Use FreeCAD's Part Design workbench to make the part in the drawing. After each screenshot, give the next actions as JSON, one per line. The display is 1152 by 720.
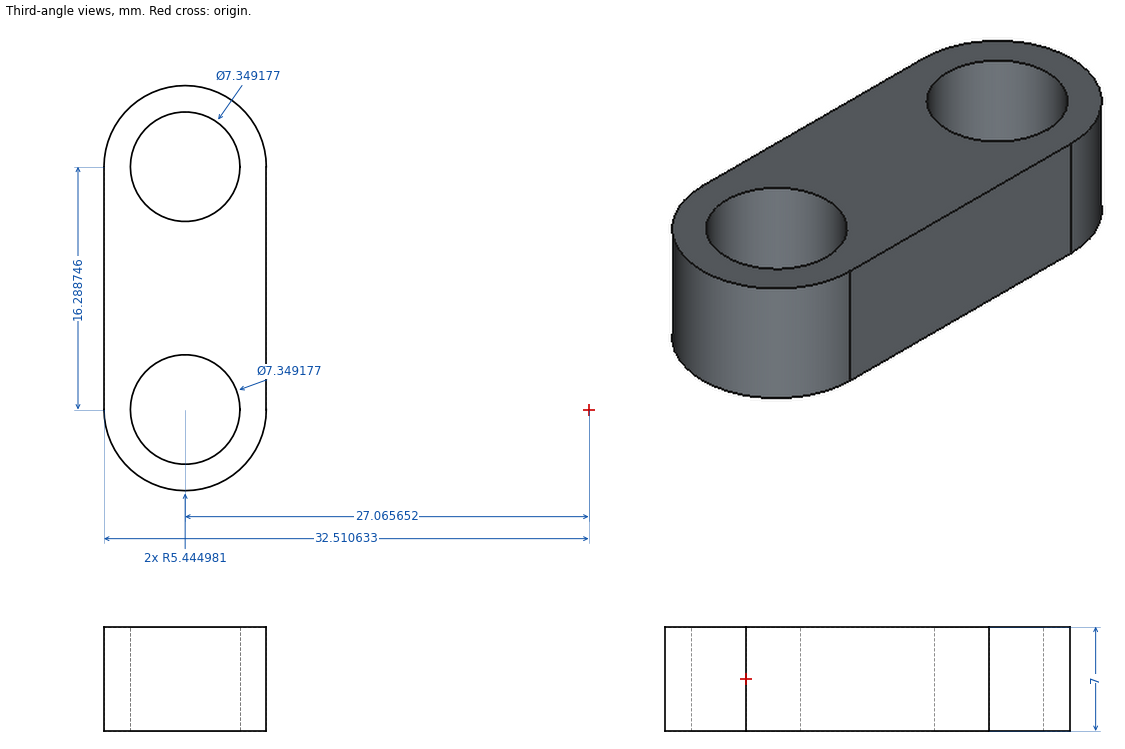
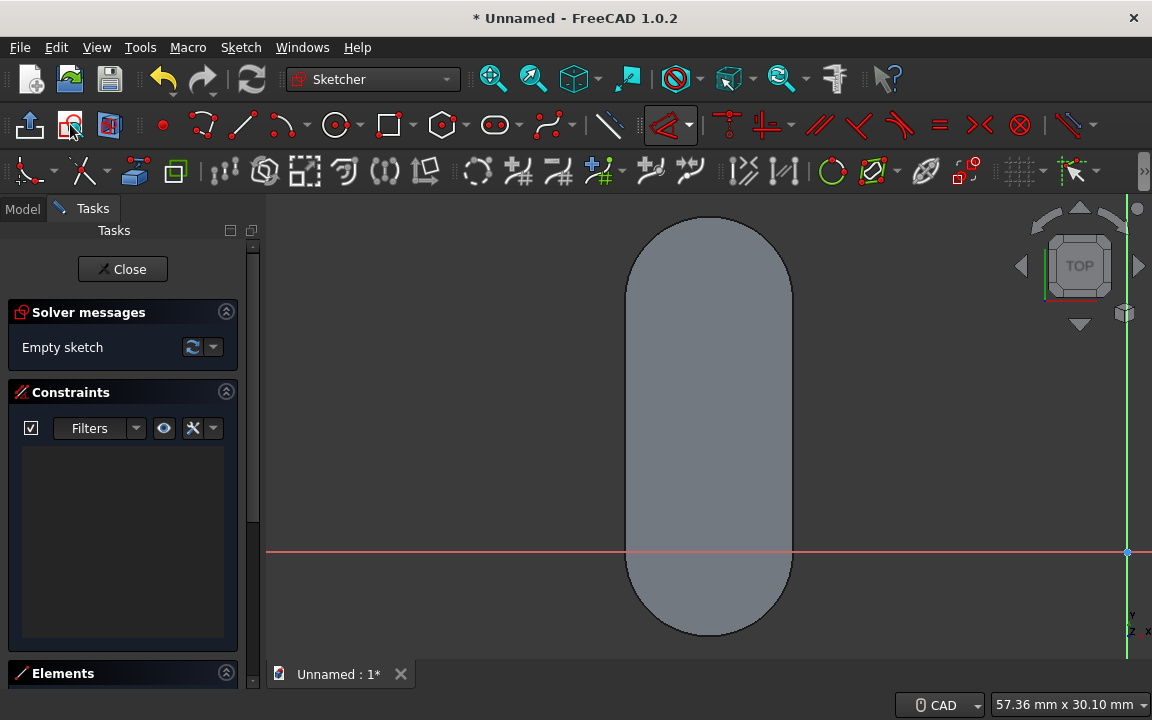
{"action": "scroll", "coordinate": [749, 626], "scroll_direction": "up", "scroll_amount": 5}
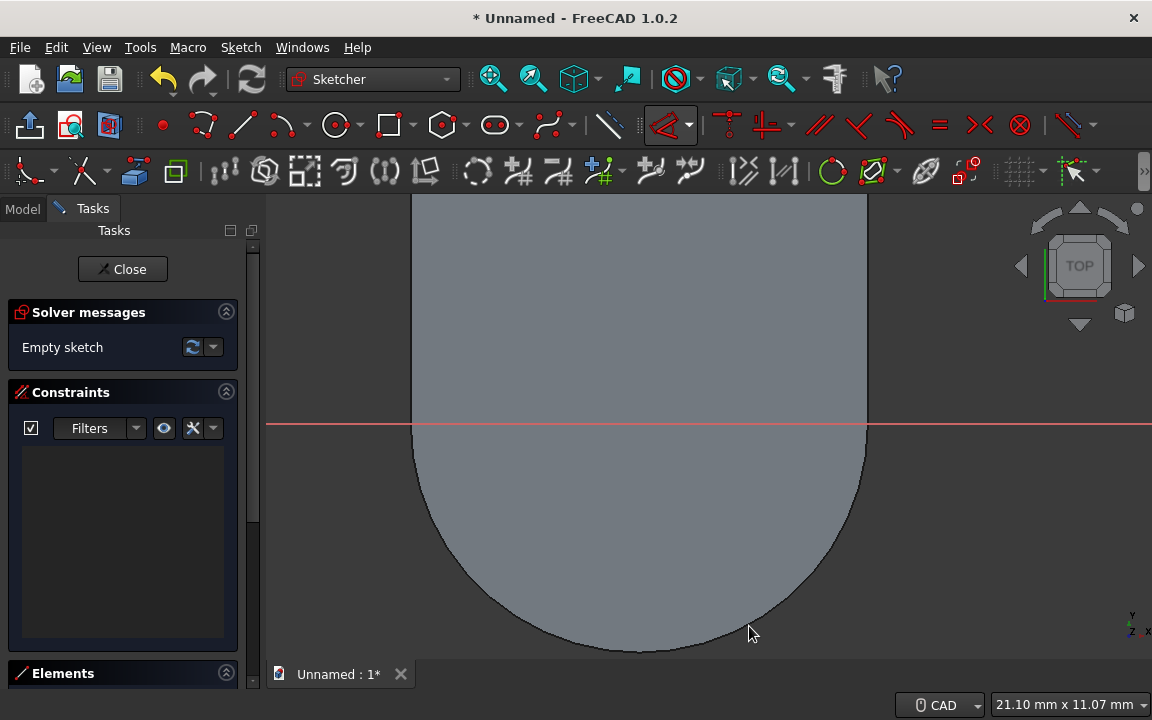
{"action": "left_click", "coordinate": [336, 126]}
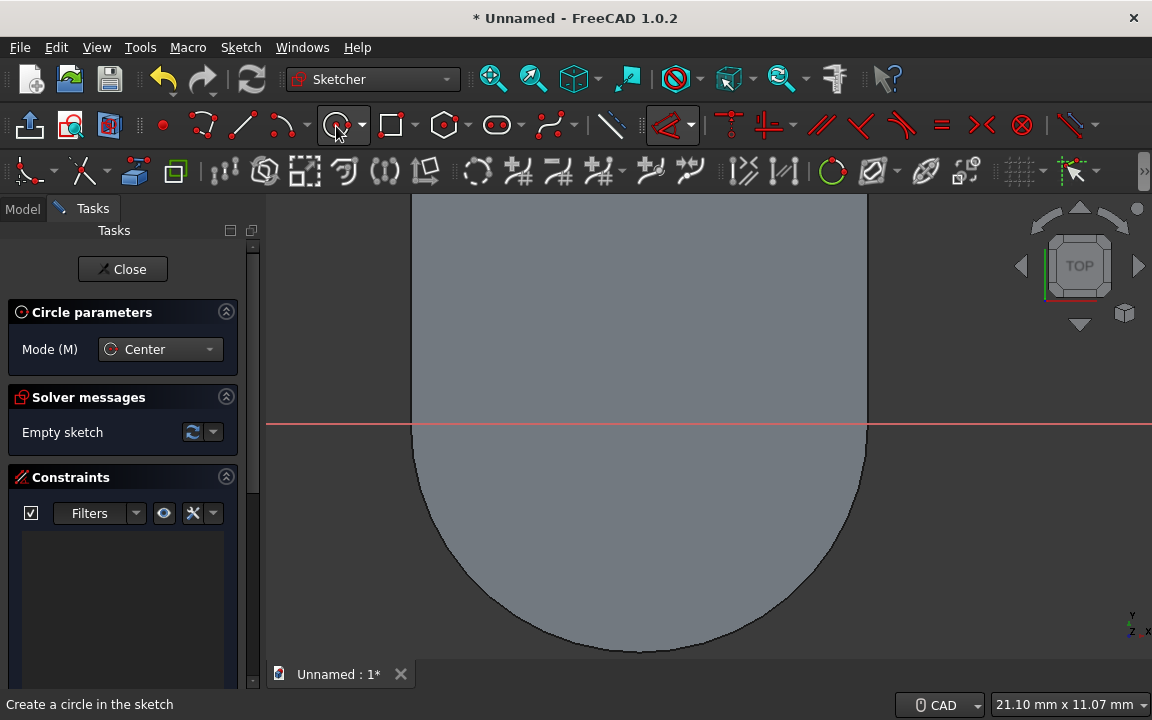
{"action": "left_click", "coordinate": [639, 424]}
{"action": "mouse_move", "coordinate": [748, 315]}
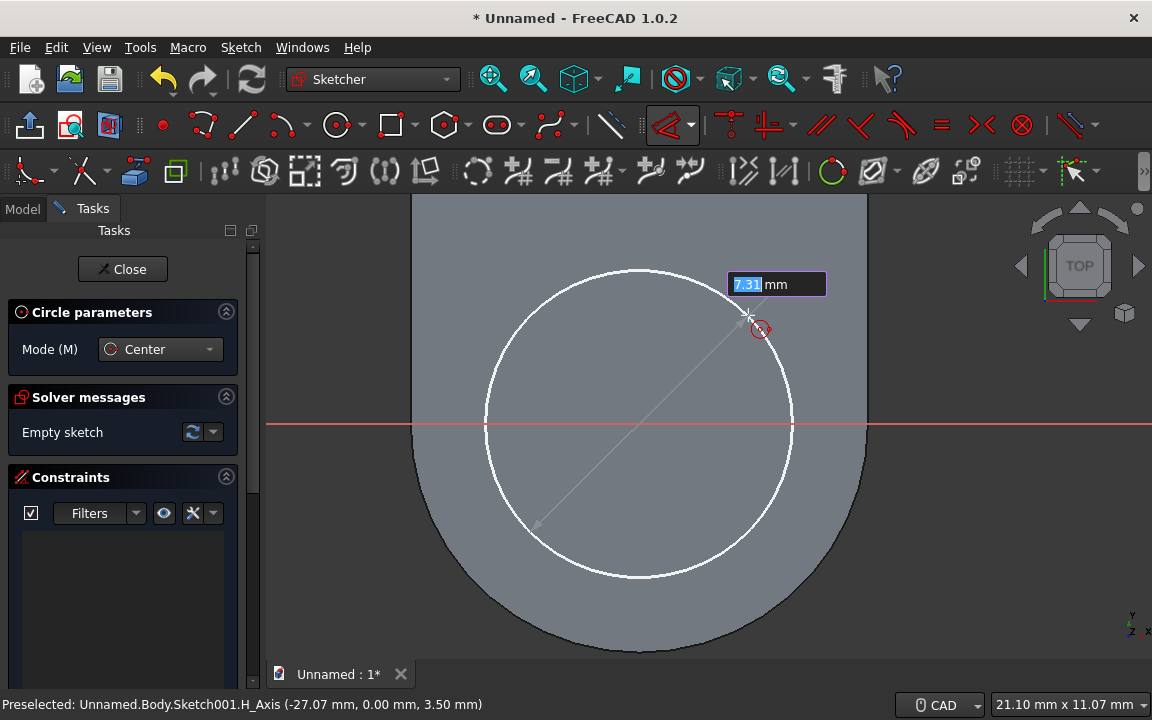
{"action": "type", "text": "7.349177"}
{"action": "key", "text": "Return"}
{"action": "key", "text": "Escape"}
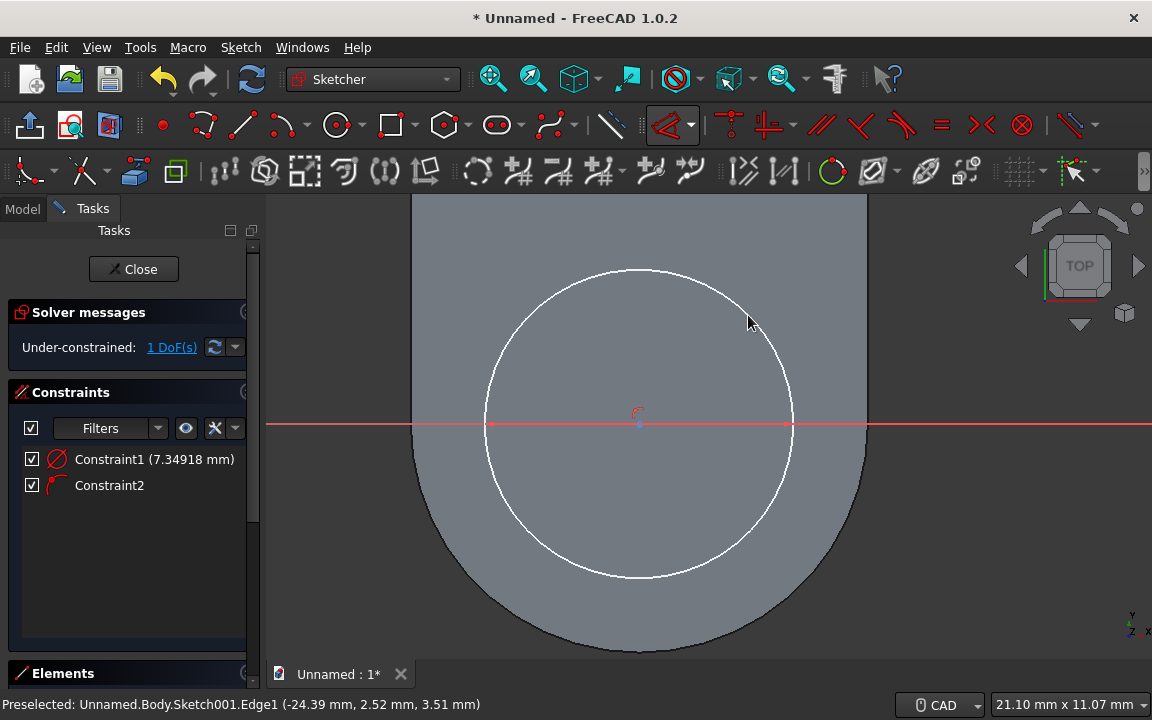
{"action": "left_click", "coordinate": [666, 126]}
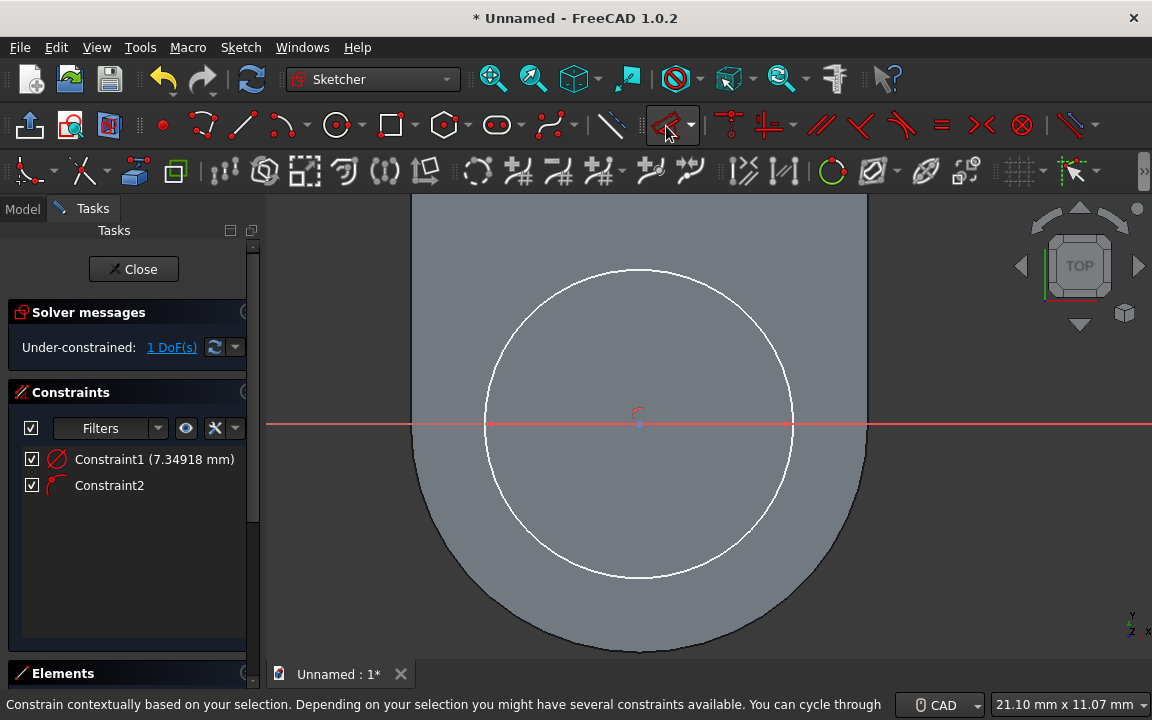
{"action": "left_click", "coordinate": [639, 424]}
{"action": "left_click", "coordinate": [813, 458]}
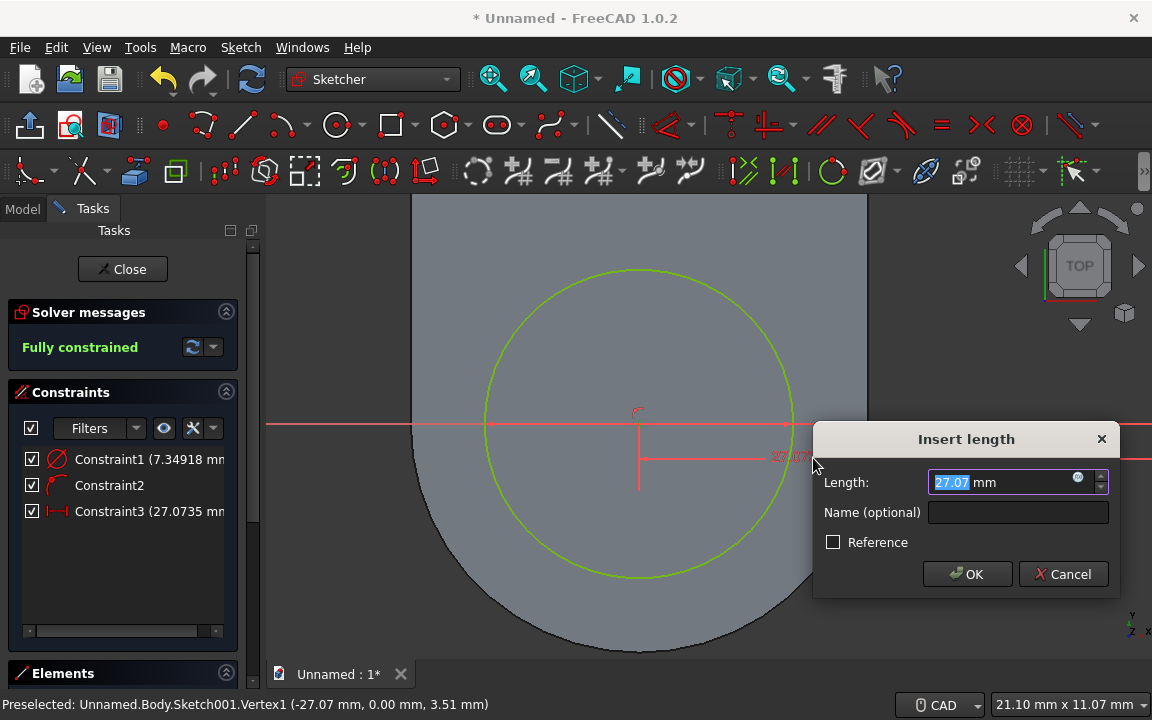
{"action": "type", "text": "27.065652"}
{"action": "key", "text": "Return"}
{"action": "key", "text": "Escape"}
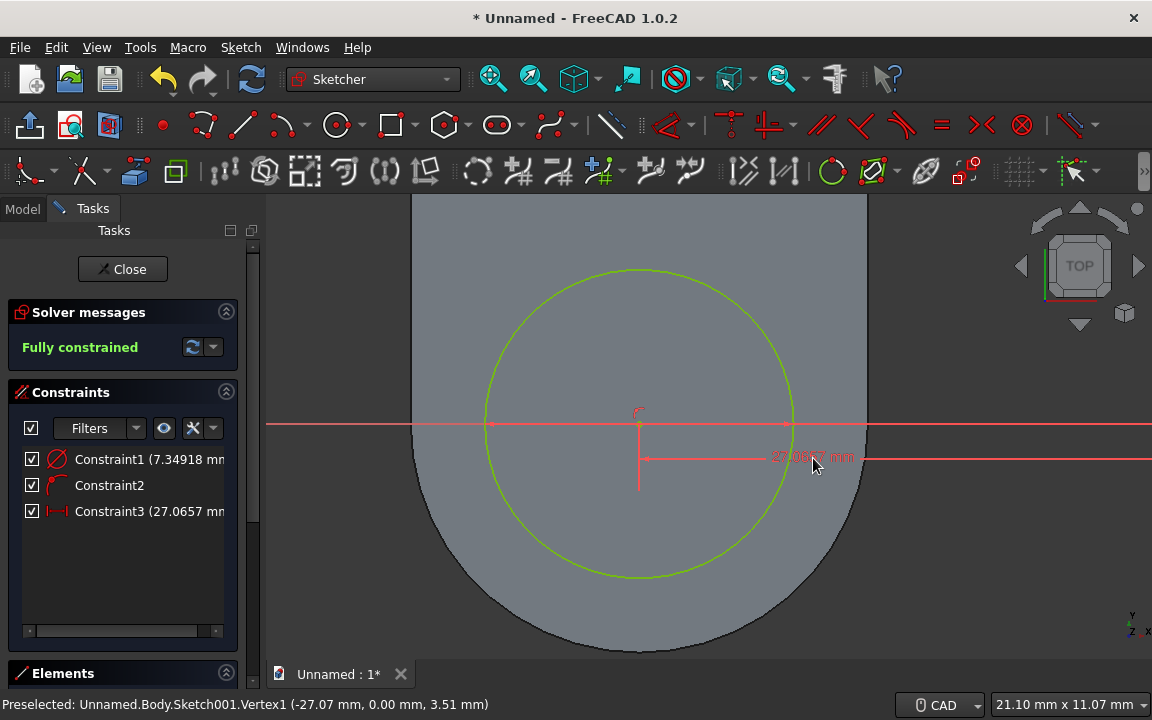
{"action": "left_click", "coordinate": [123, 269]}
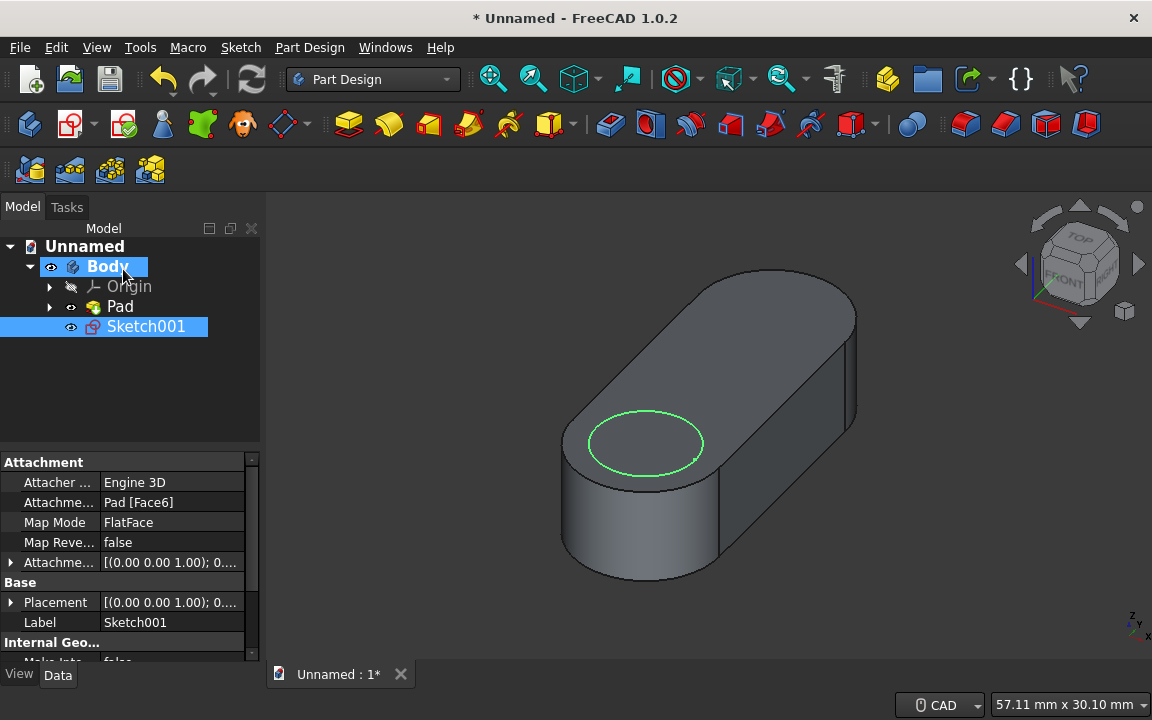
{"action": "left_click", "coordinate": [612, 124]}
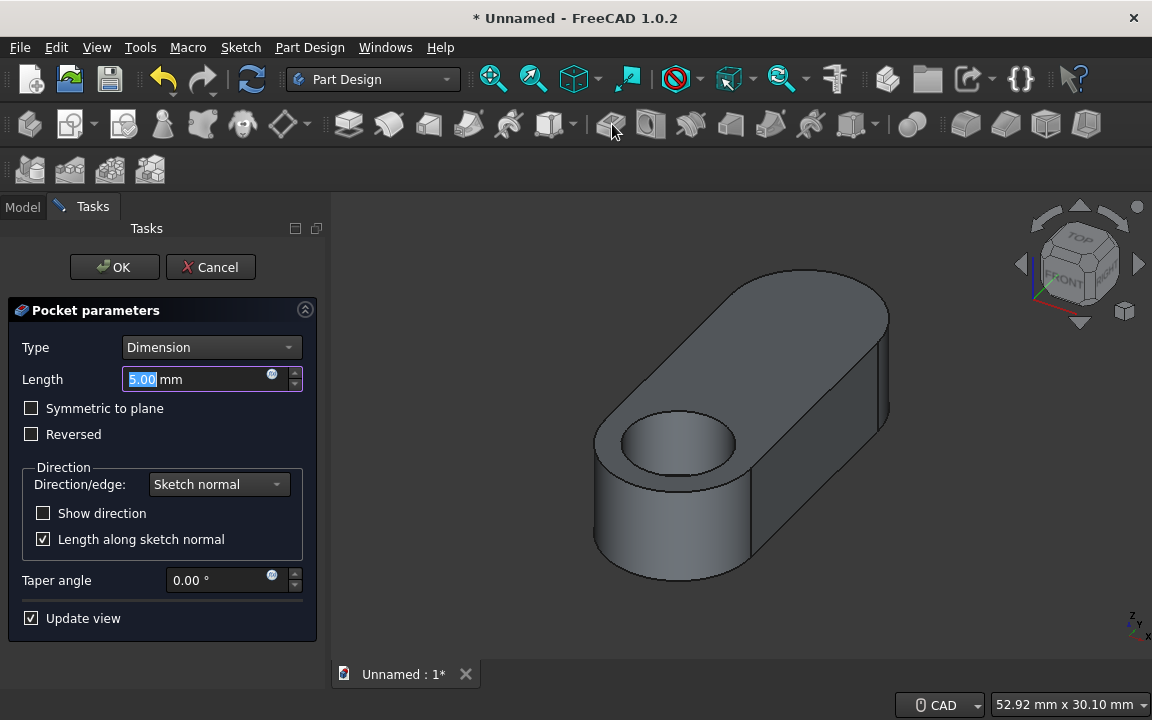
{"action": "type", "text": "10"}
{"action": "key", "text": "Tab"}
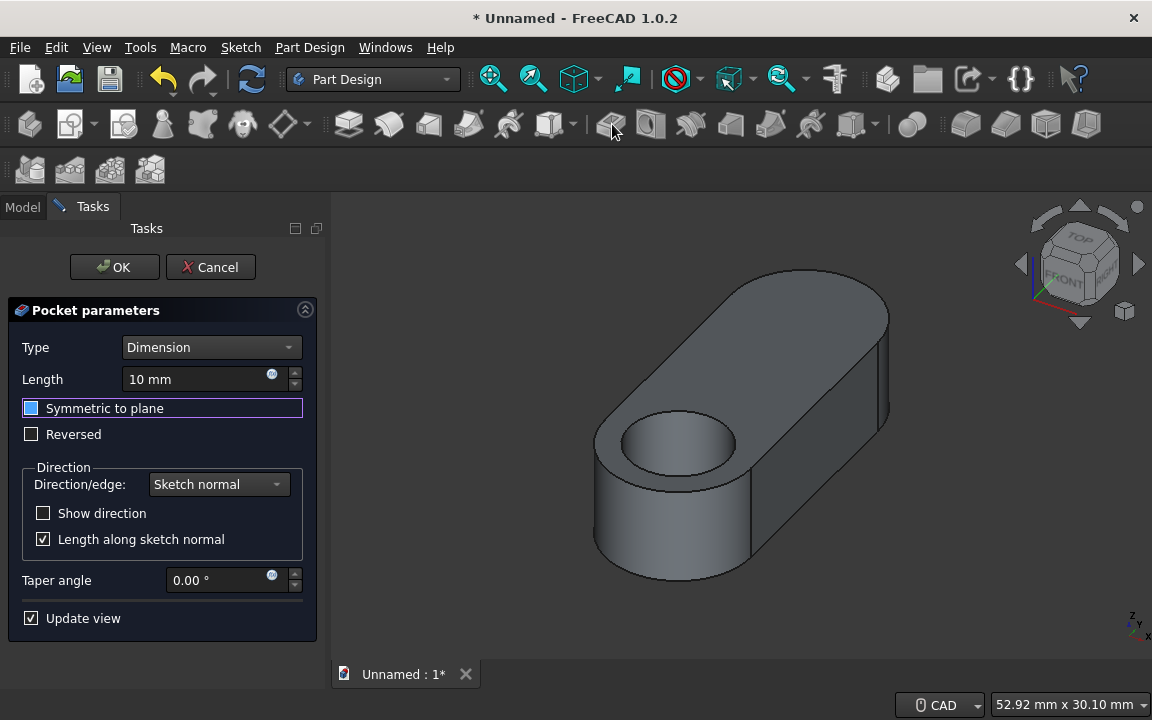
{"action": "left_click", "coordinate": [115, 267]}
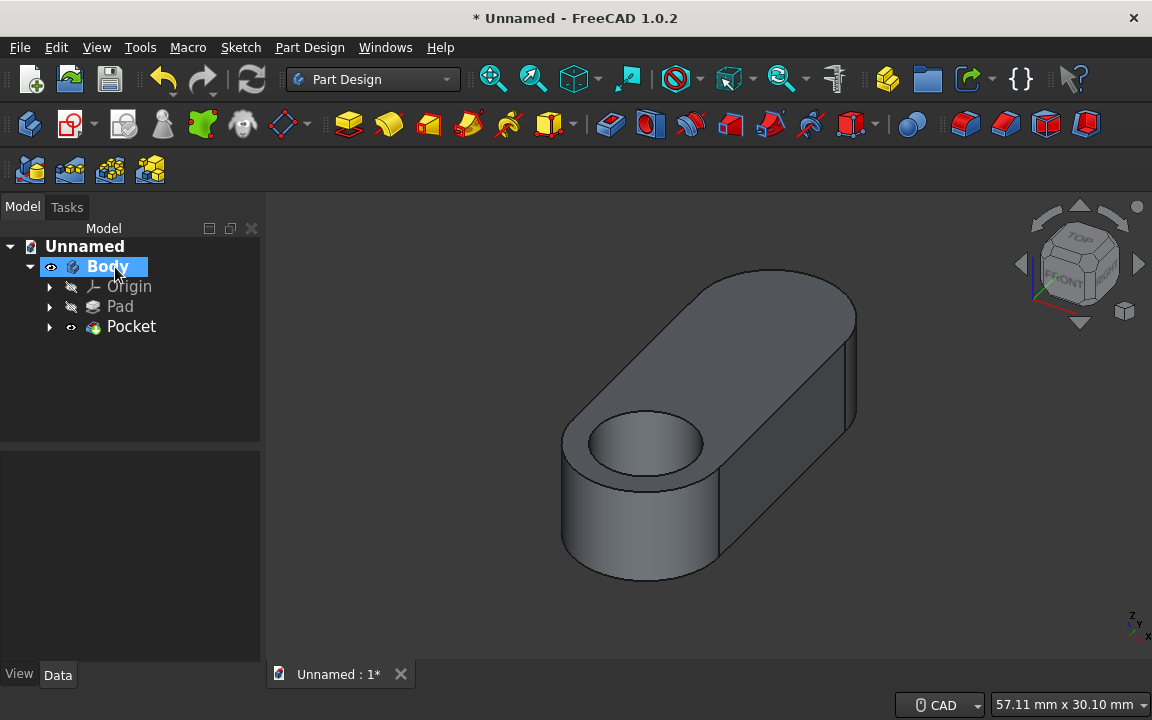
{"action": "left_click", "coordinate": [769, 320]}